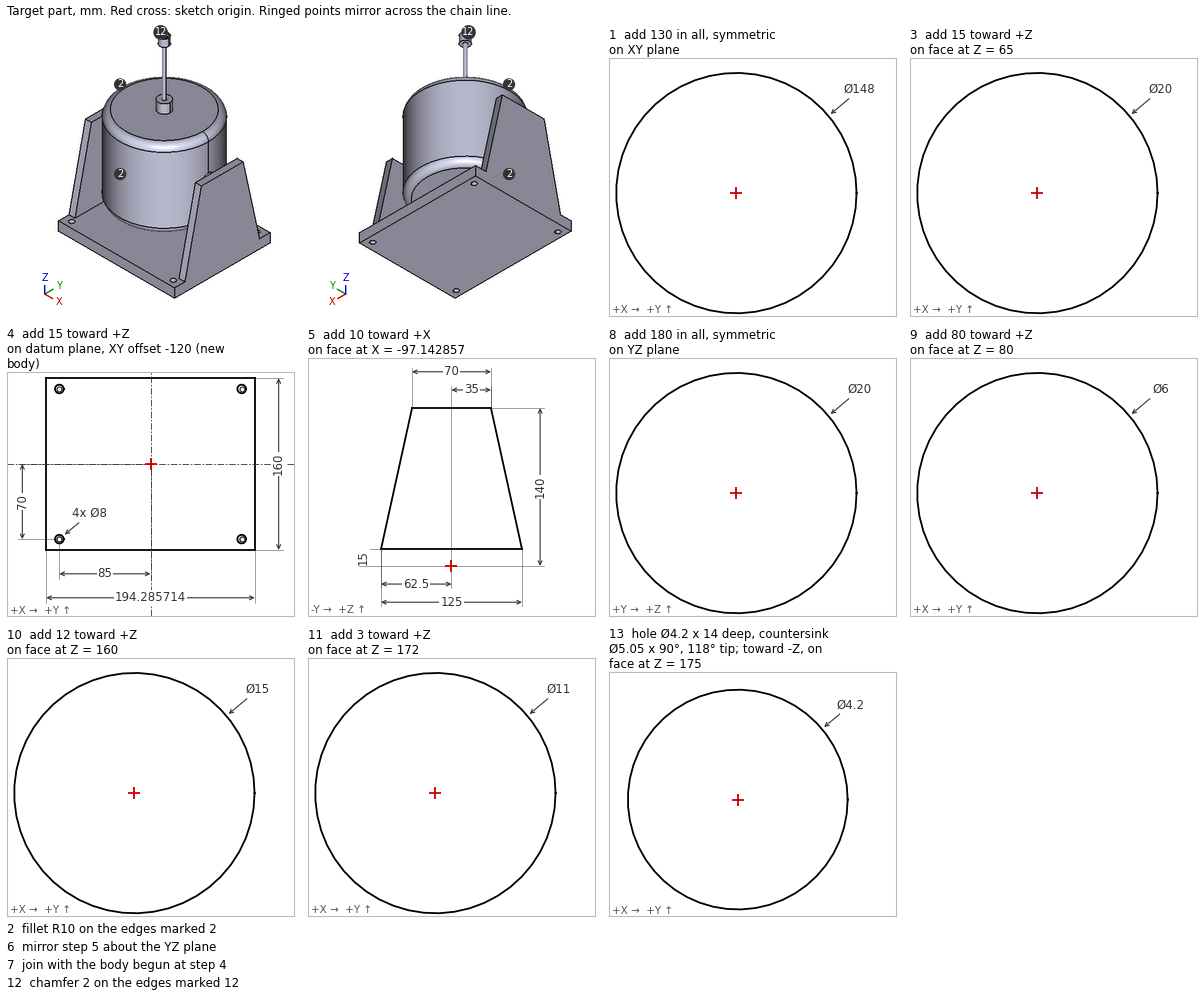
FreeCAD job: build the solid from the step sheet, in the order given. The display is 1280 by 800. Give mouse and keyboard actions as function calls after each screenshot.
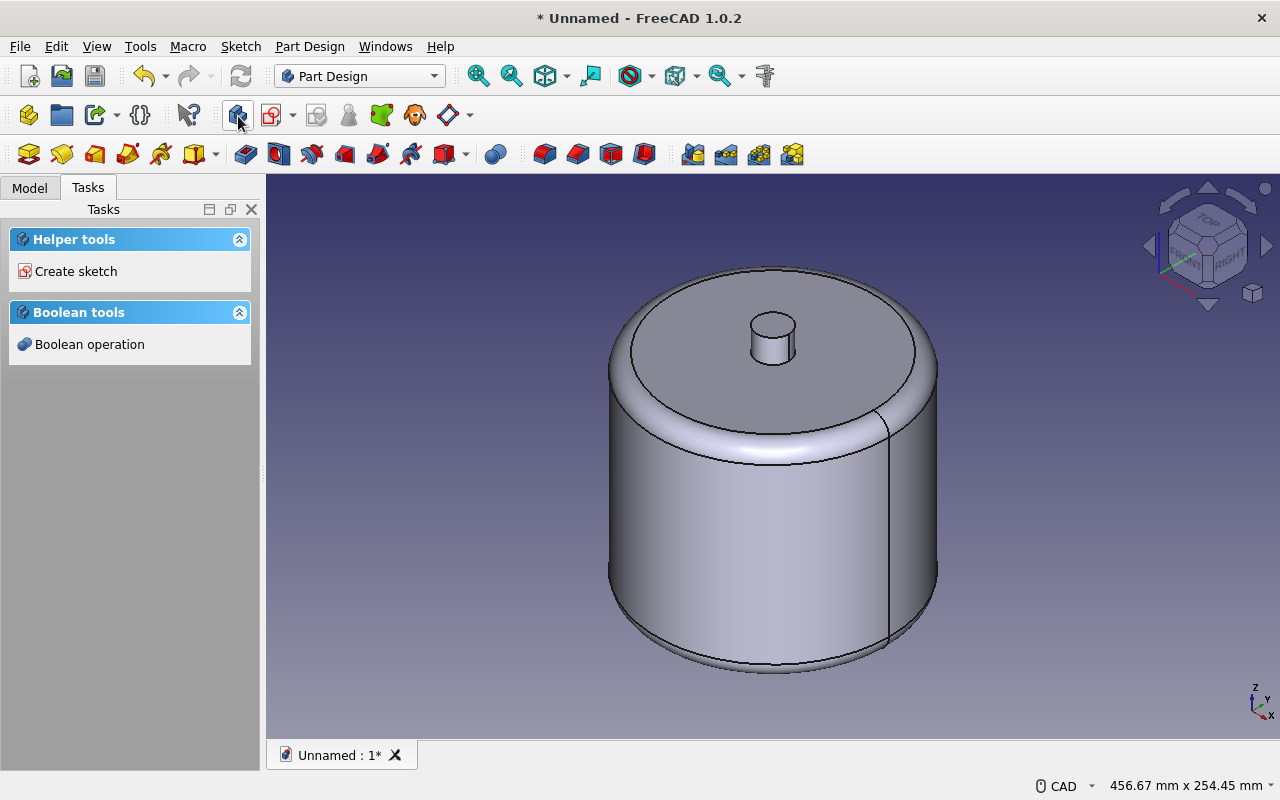
click(30, 188)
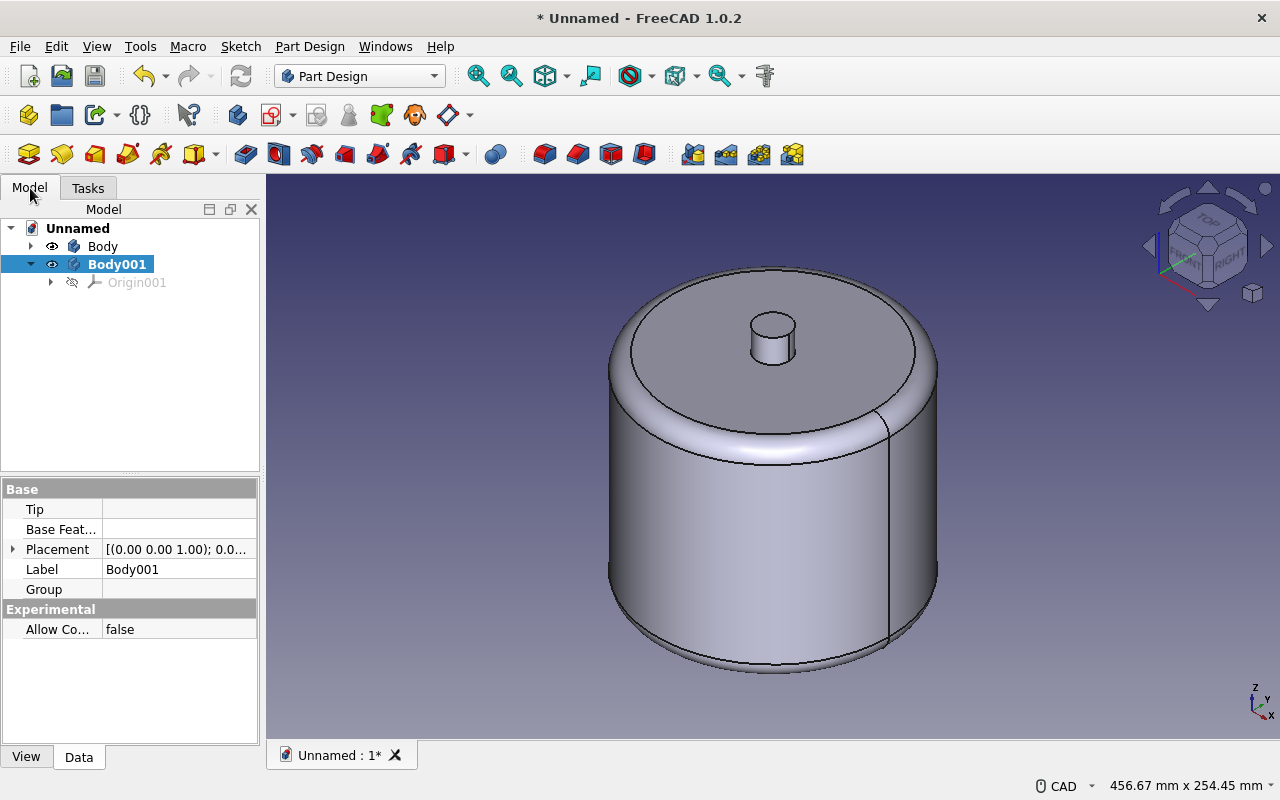
click(51, 282)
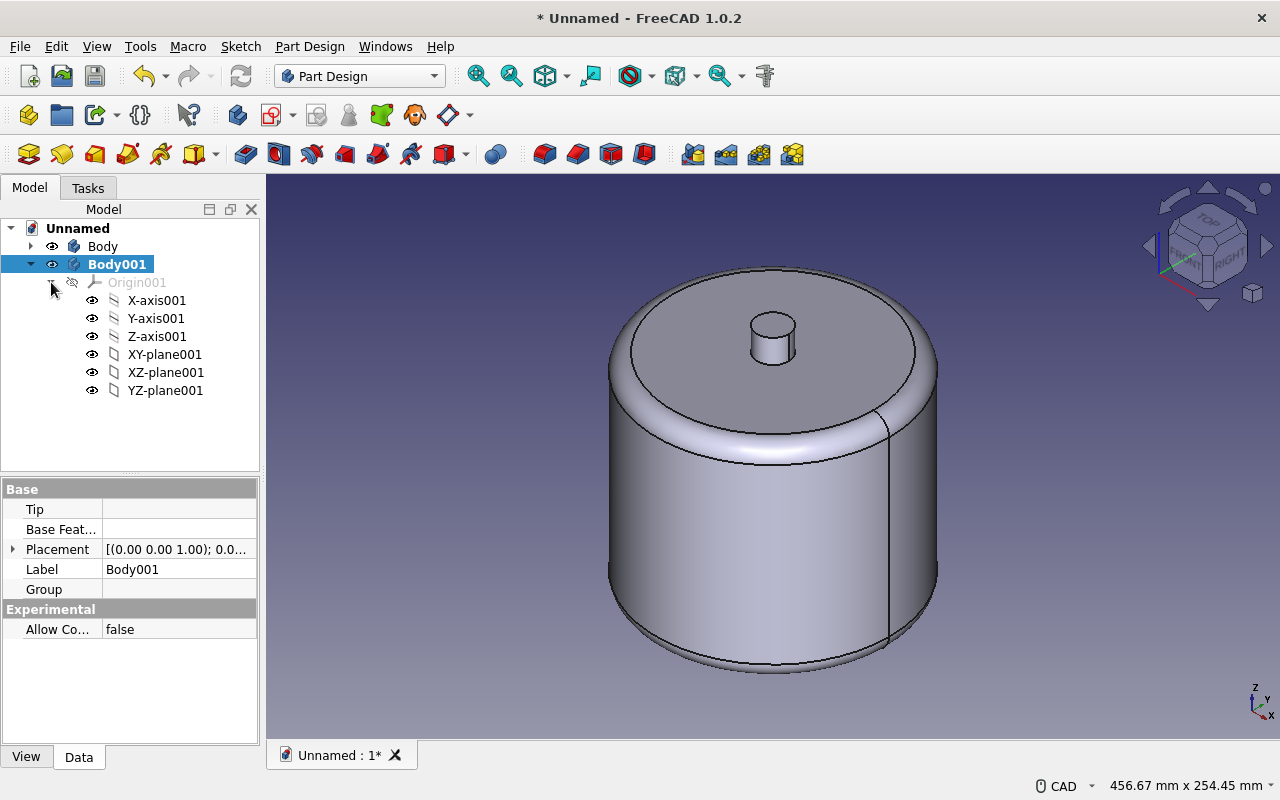
click(137, 354)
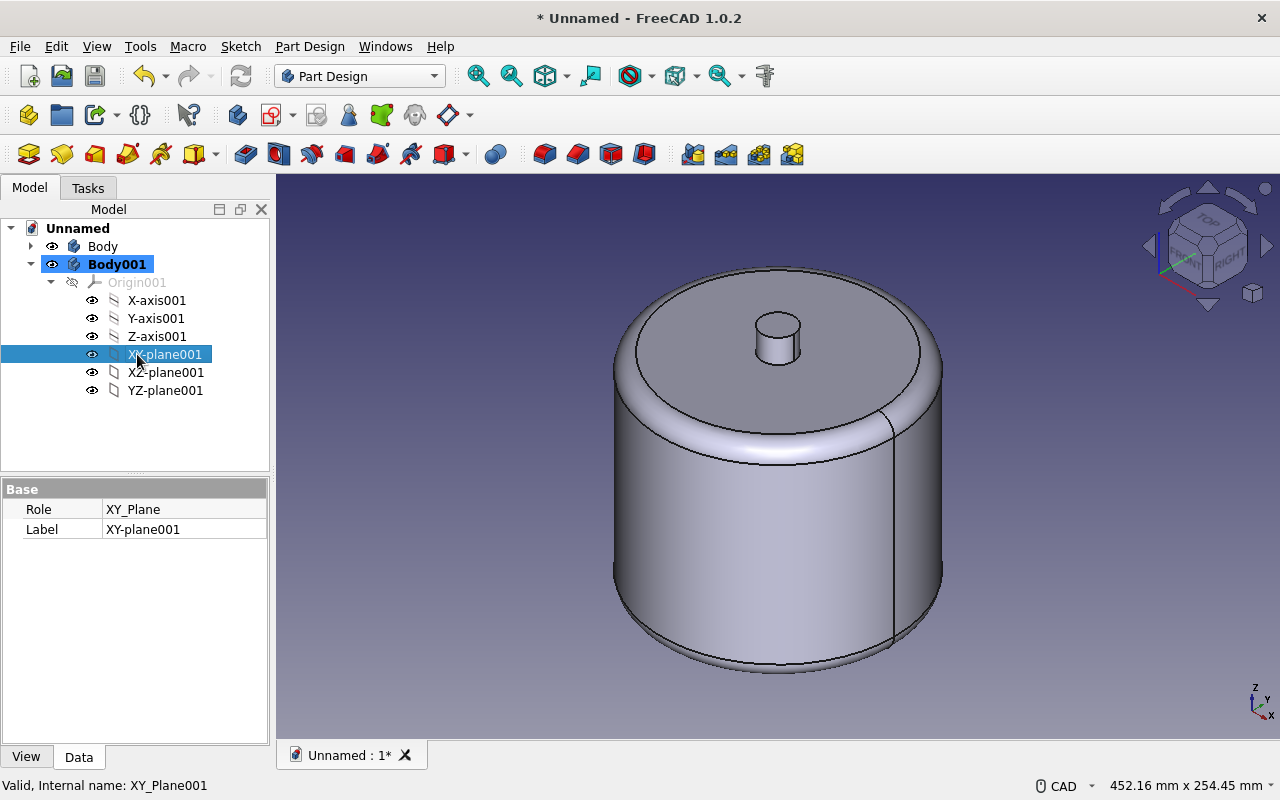
click(448, 116)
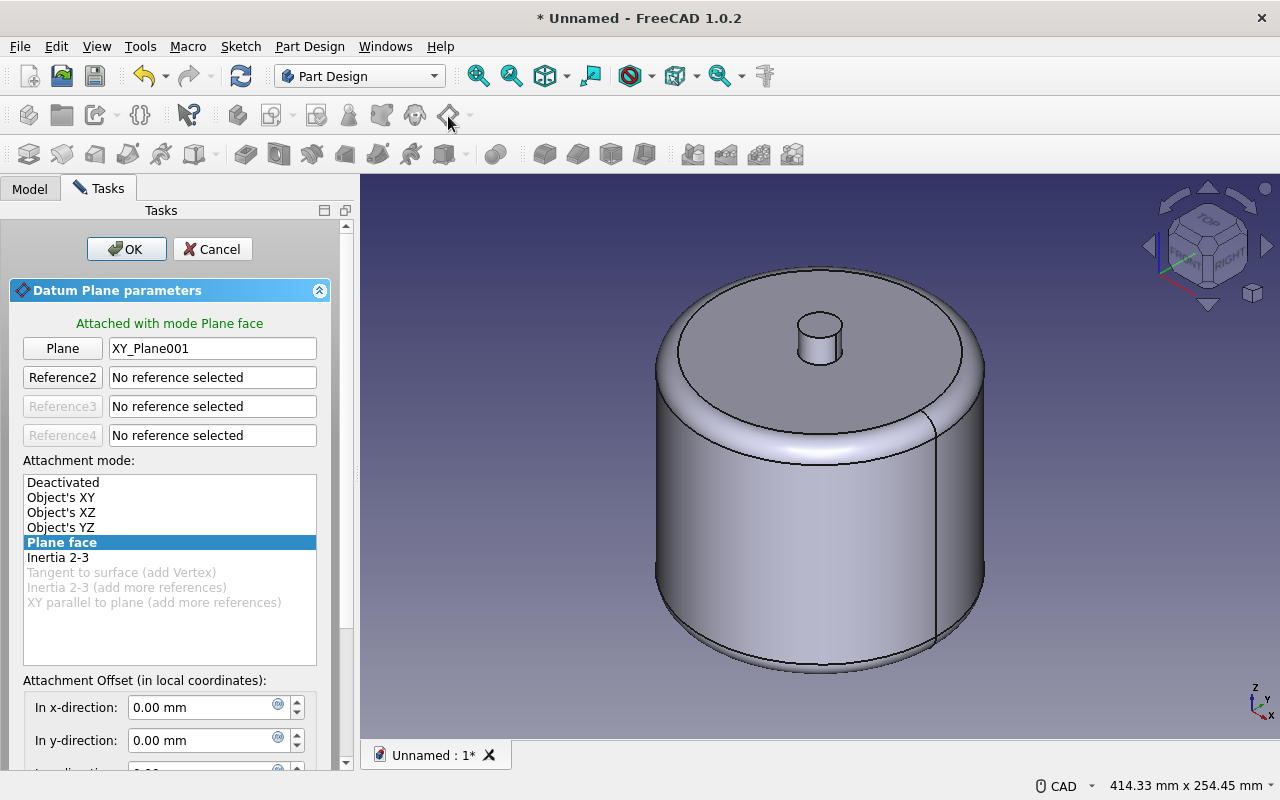
scroll(346, 495, down, 2)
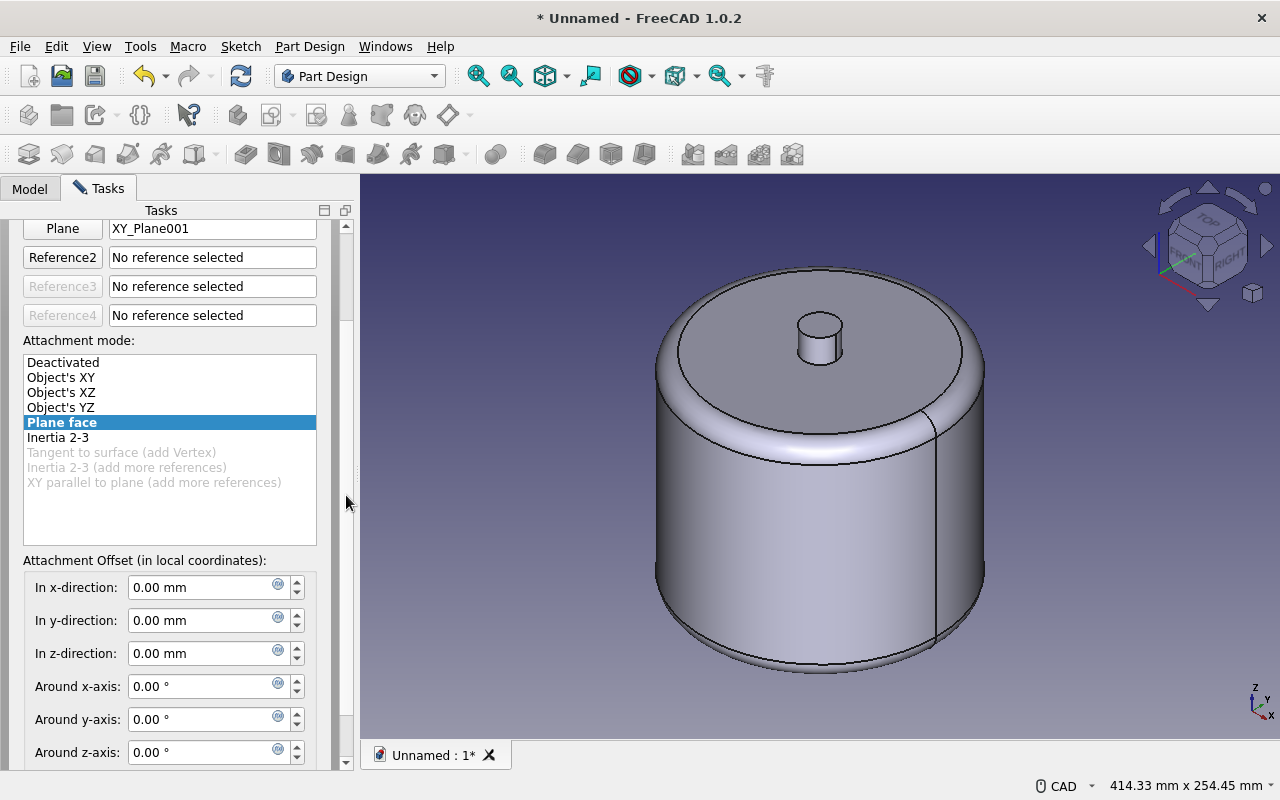
triple_click(210, 654)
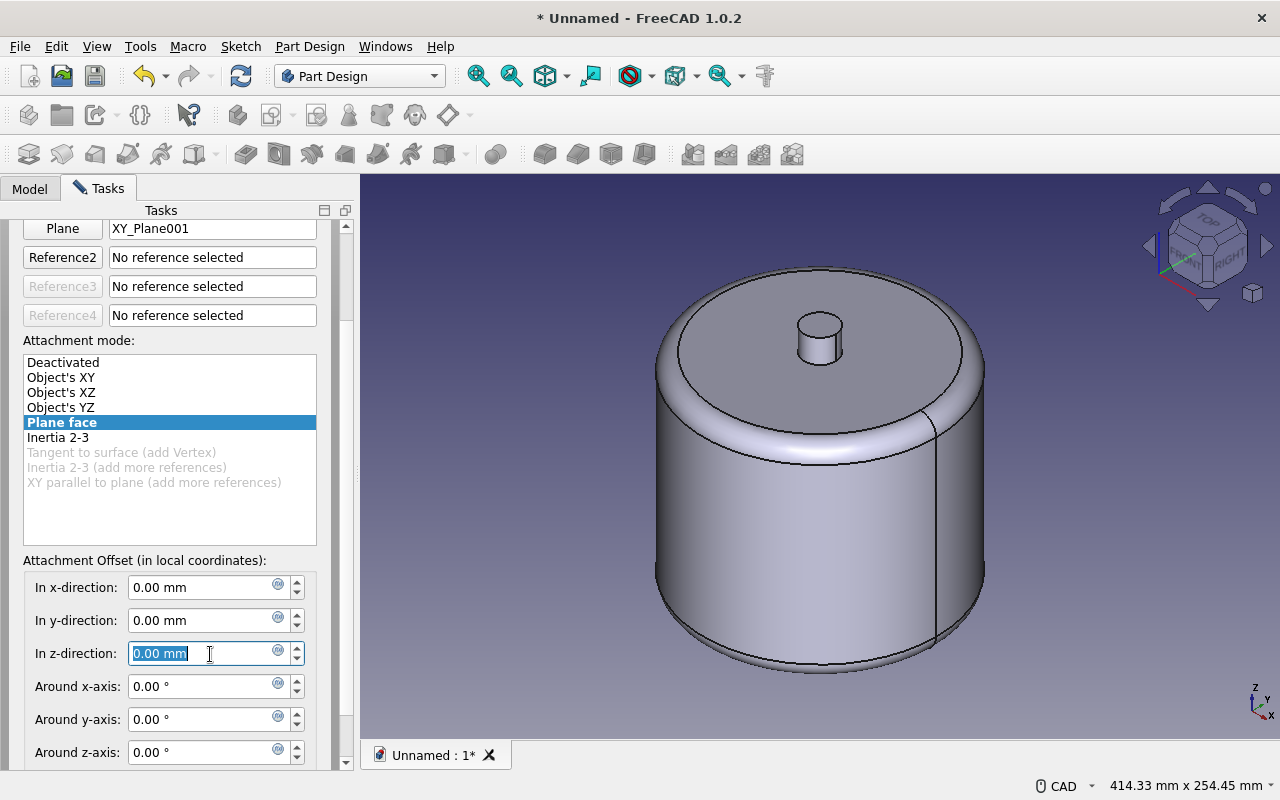
text(-120)
key(Tab)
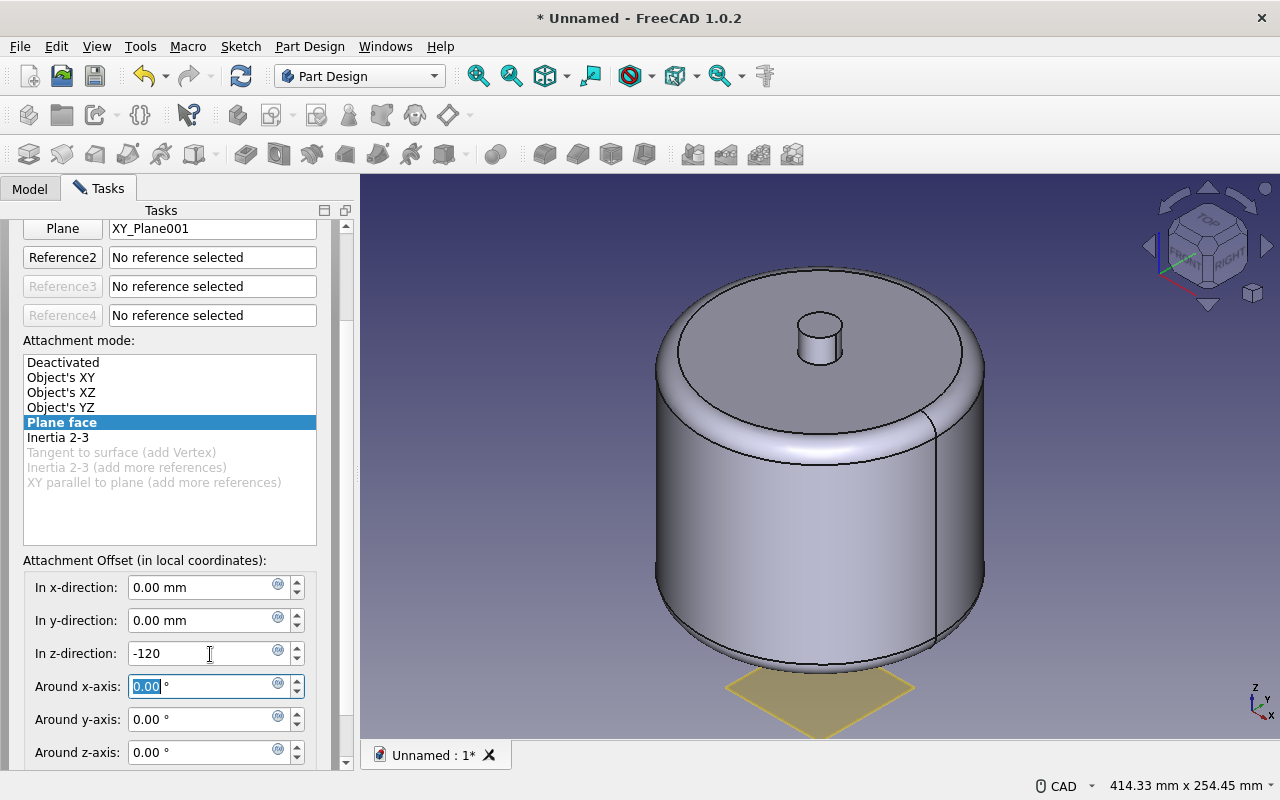
scroll(346, 495, up, 3)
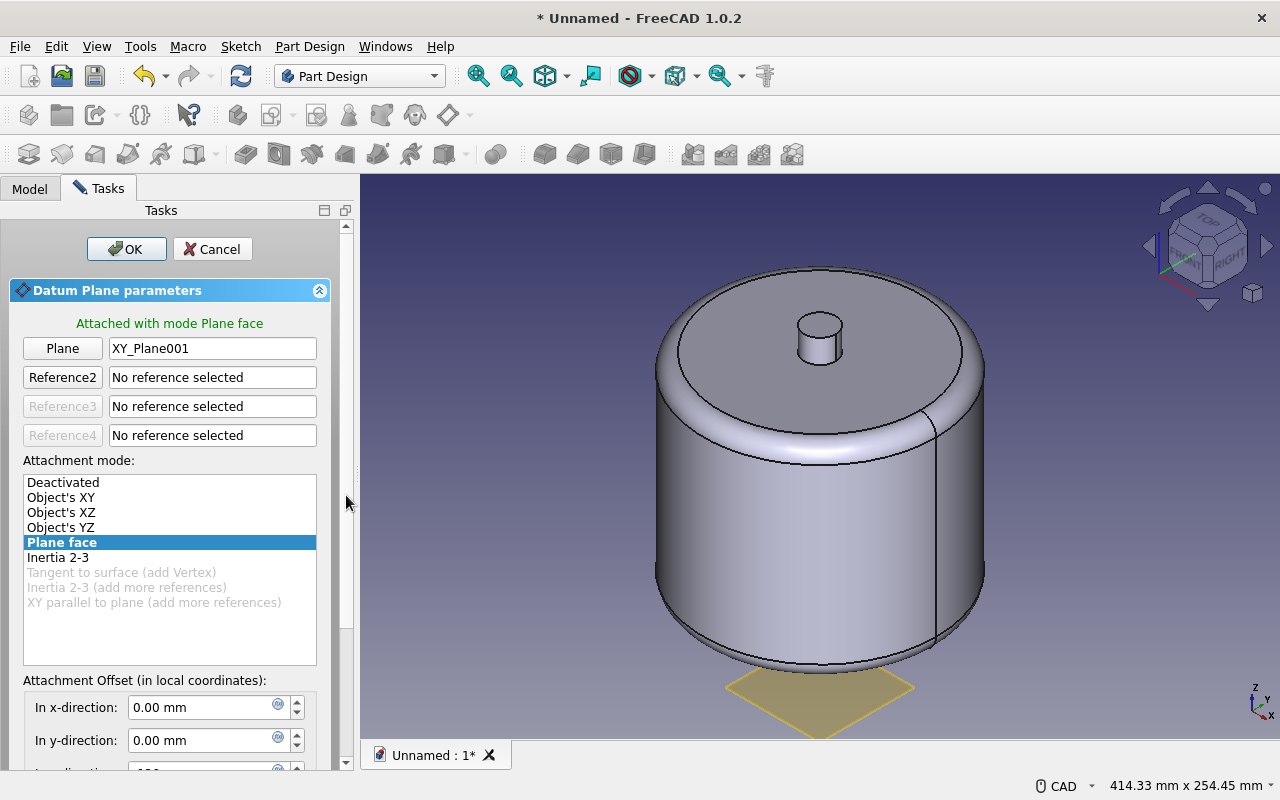
click(127, 249)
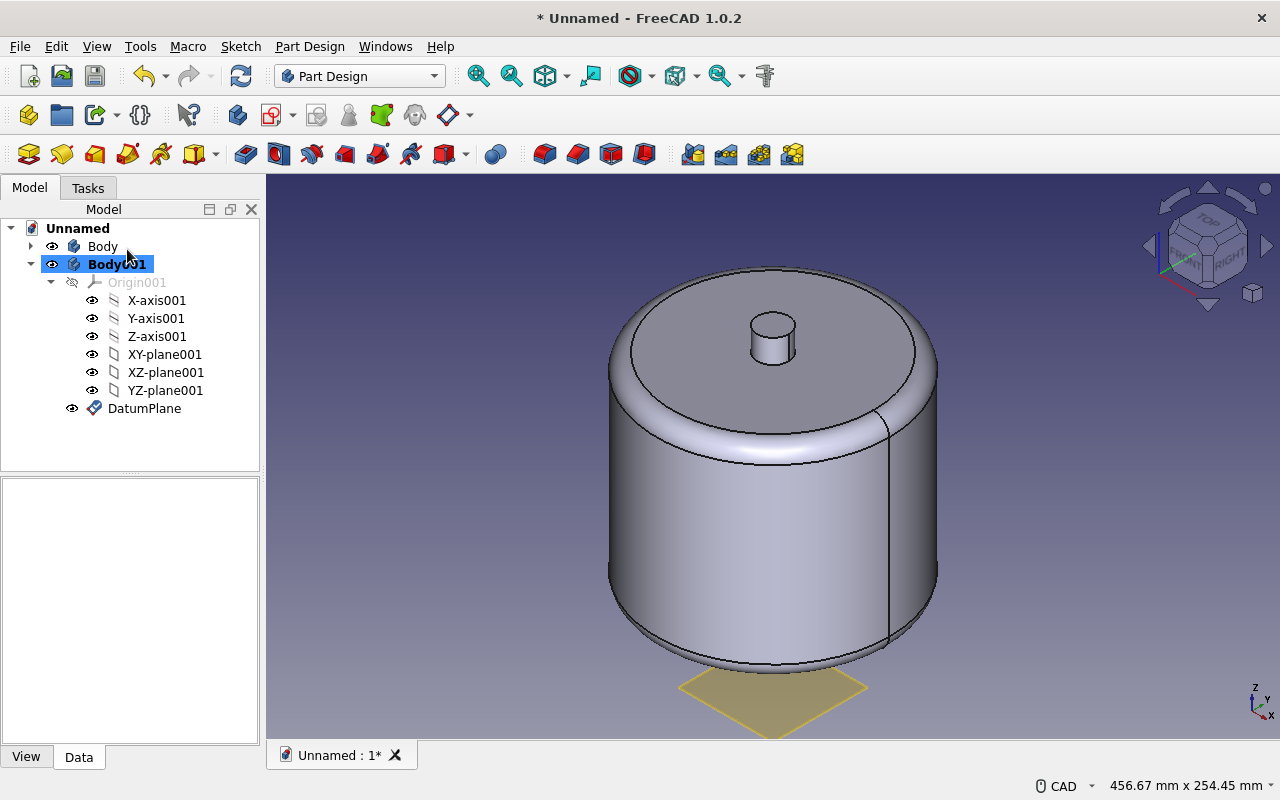
click(117, 408)